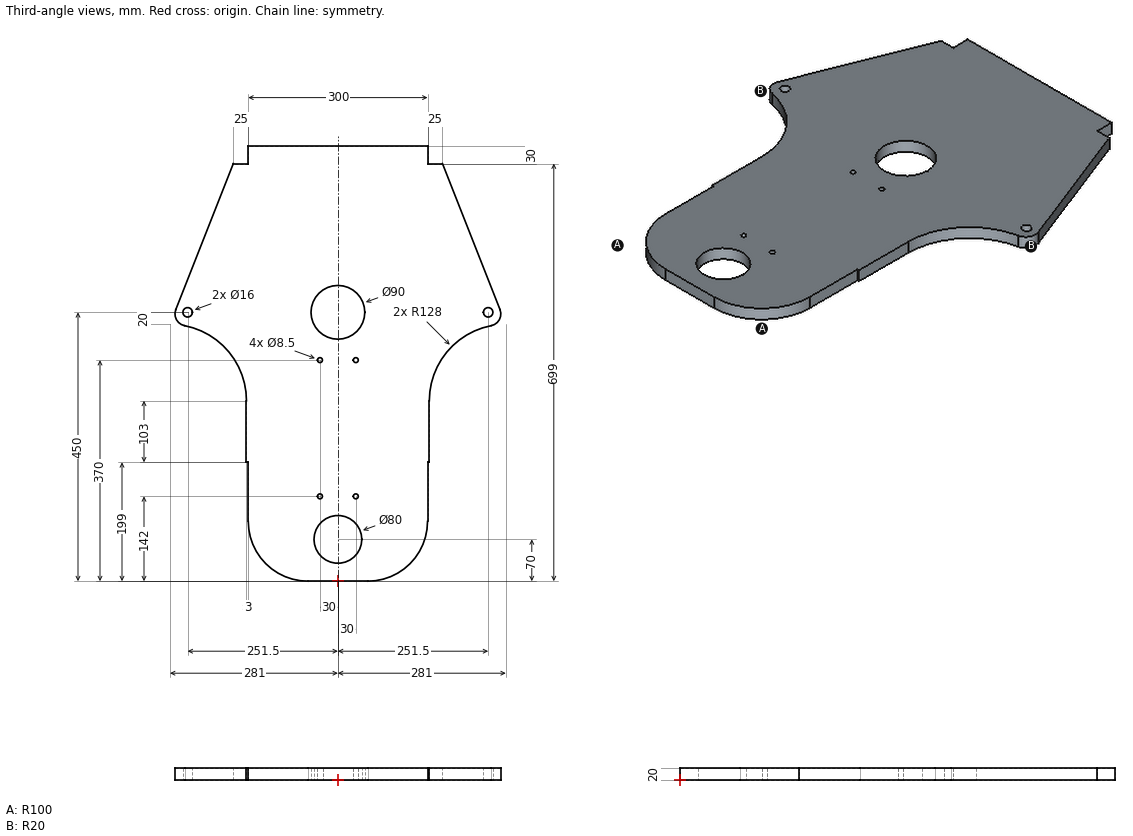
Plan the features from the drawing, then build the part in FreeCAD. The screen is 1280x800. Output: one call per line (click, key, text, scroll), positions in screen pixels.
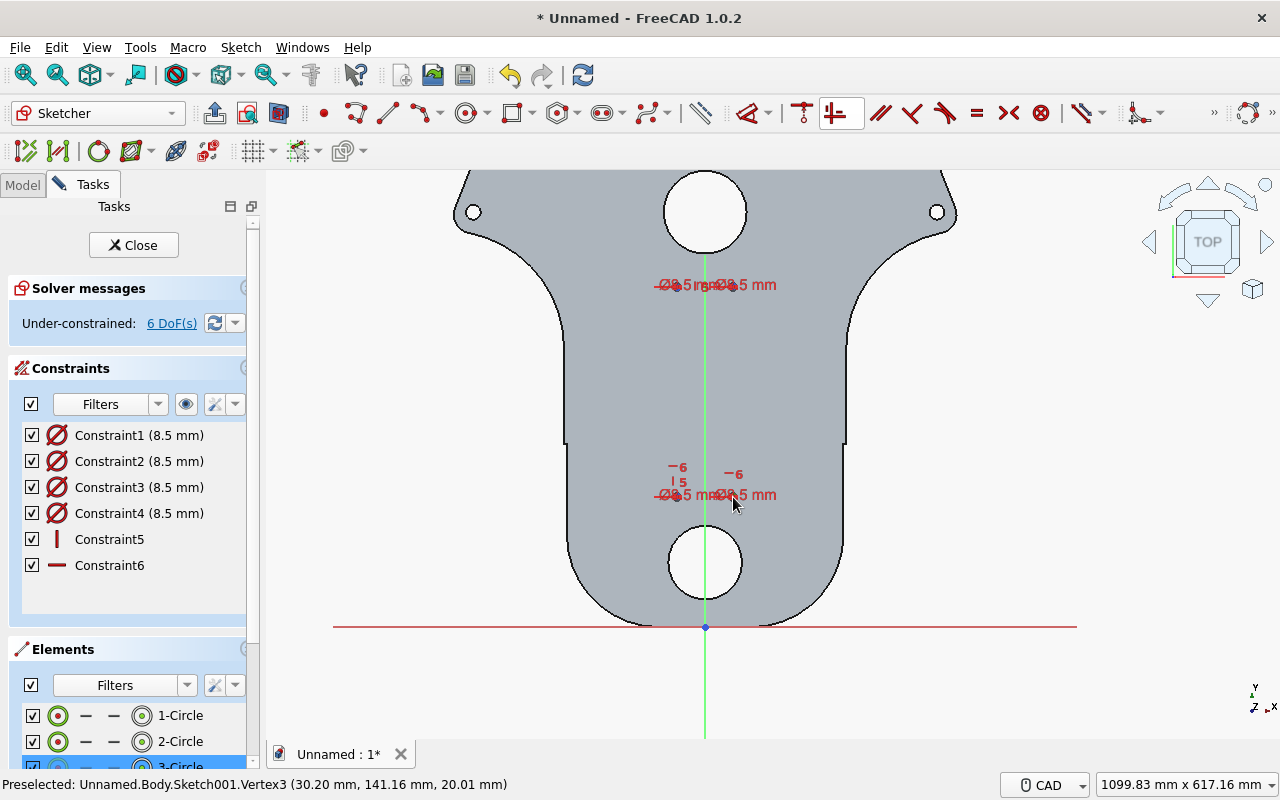
click(733, 287)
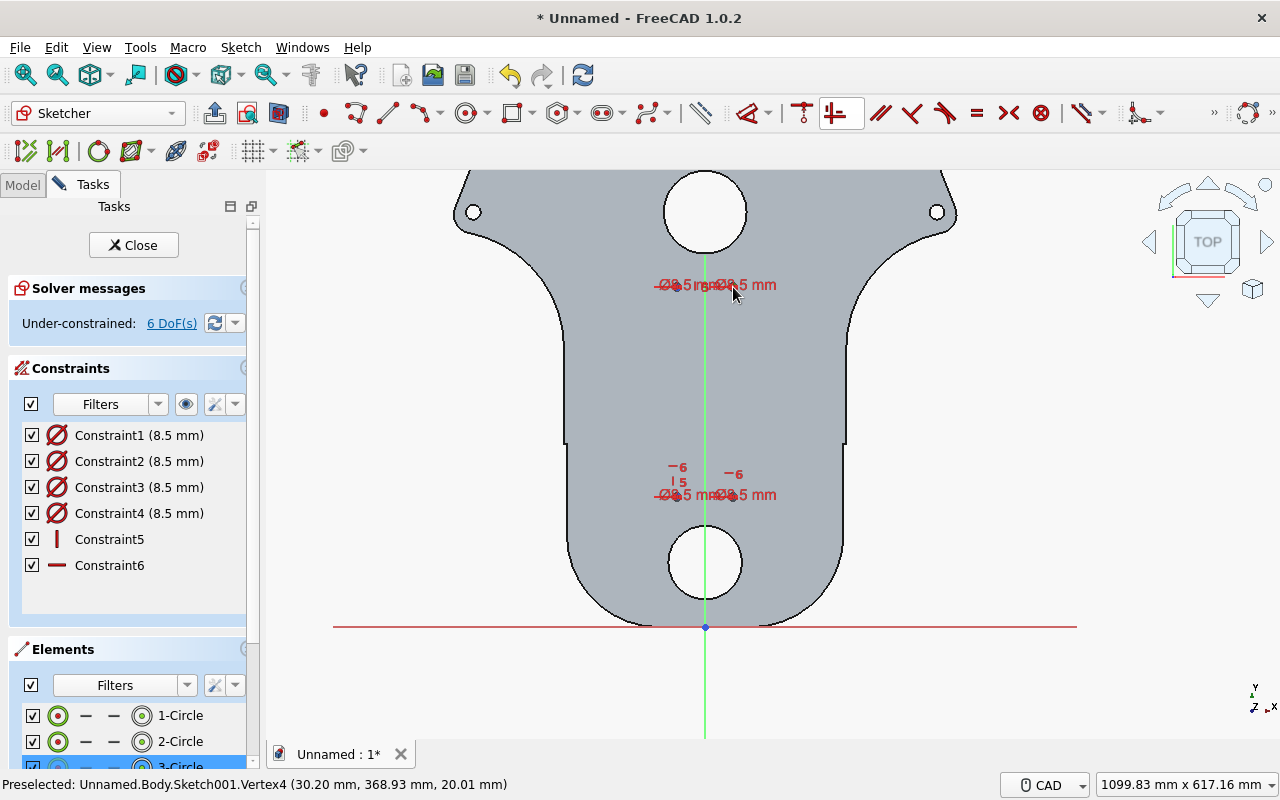
click(858, 114)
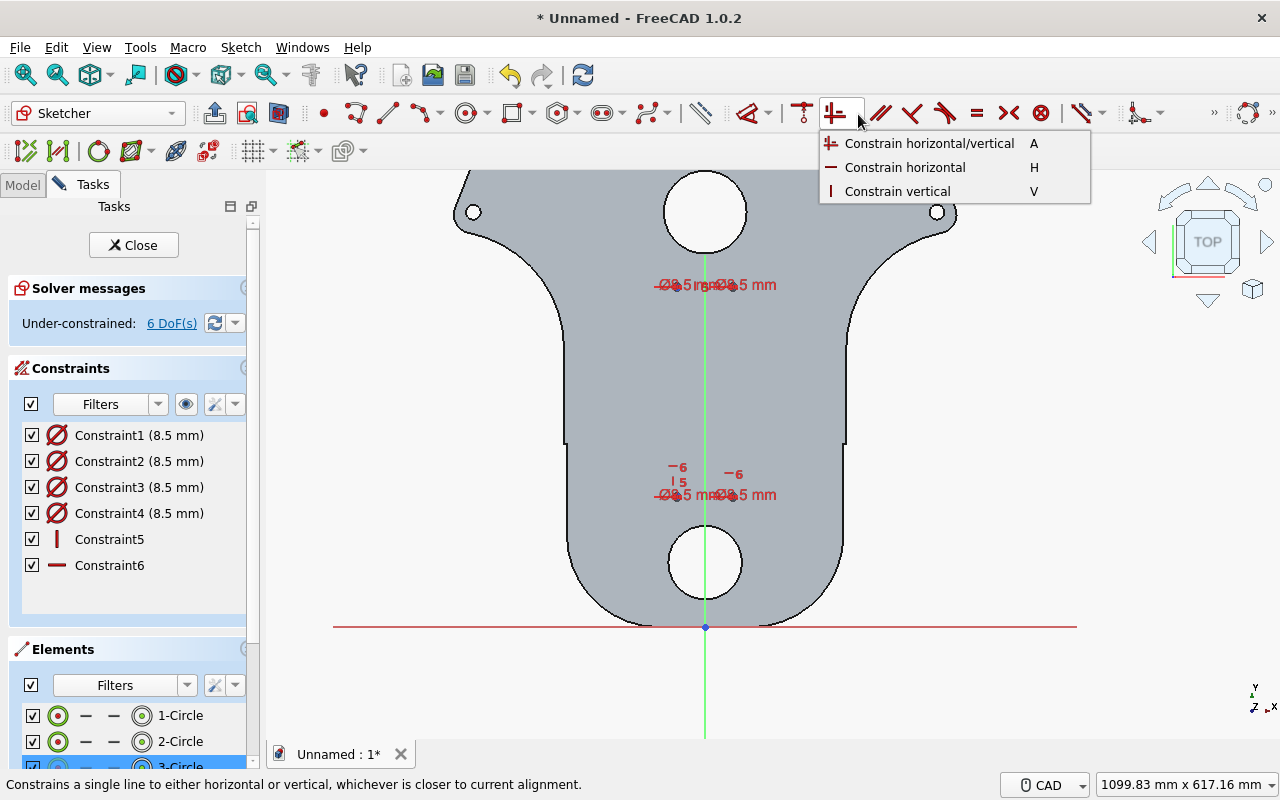
click(955, 191)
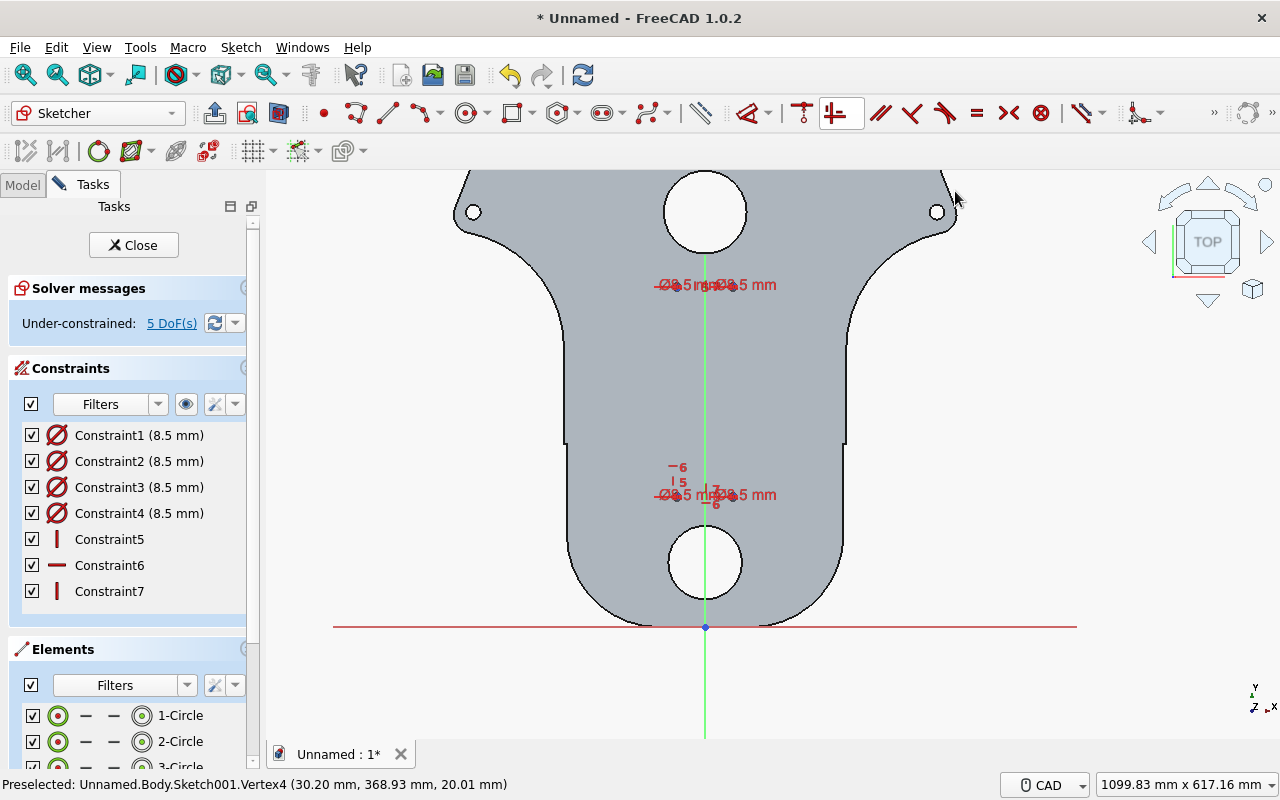
click(677, 287)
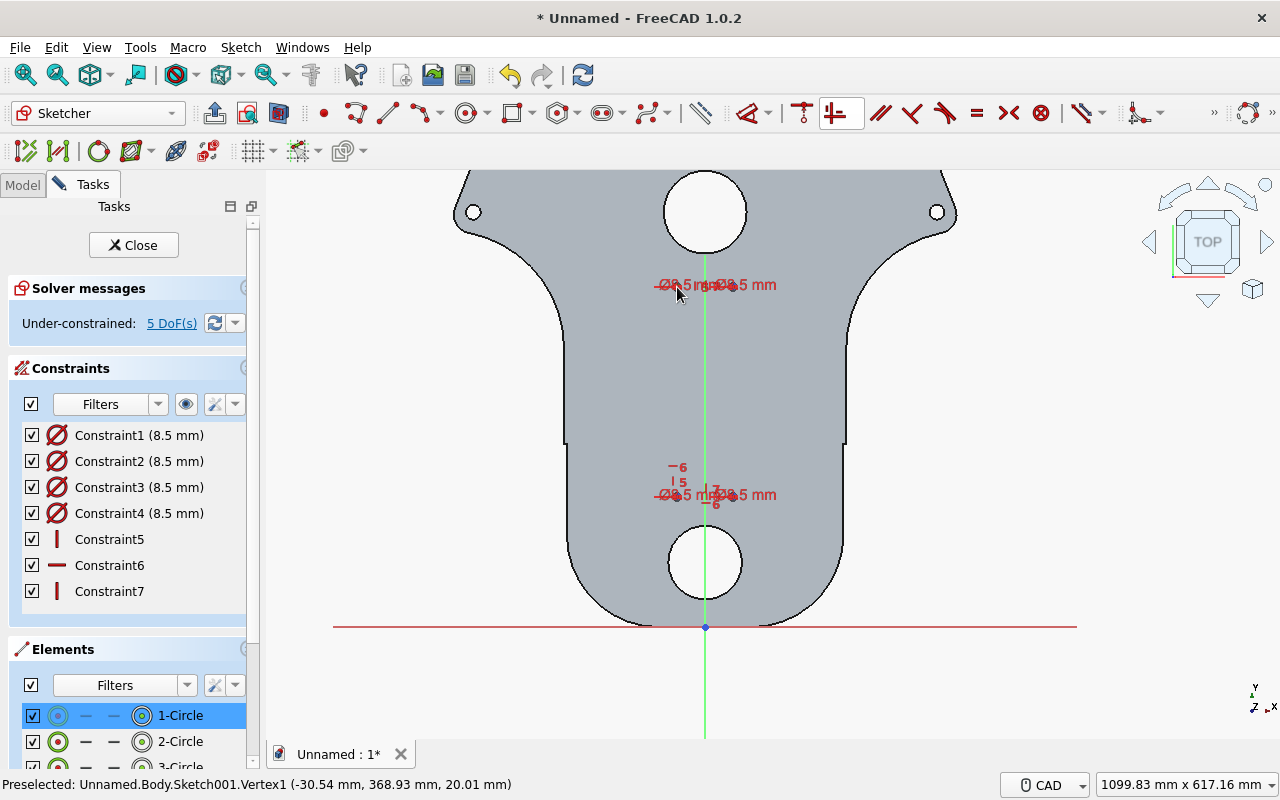
click(733, 287)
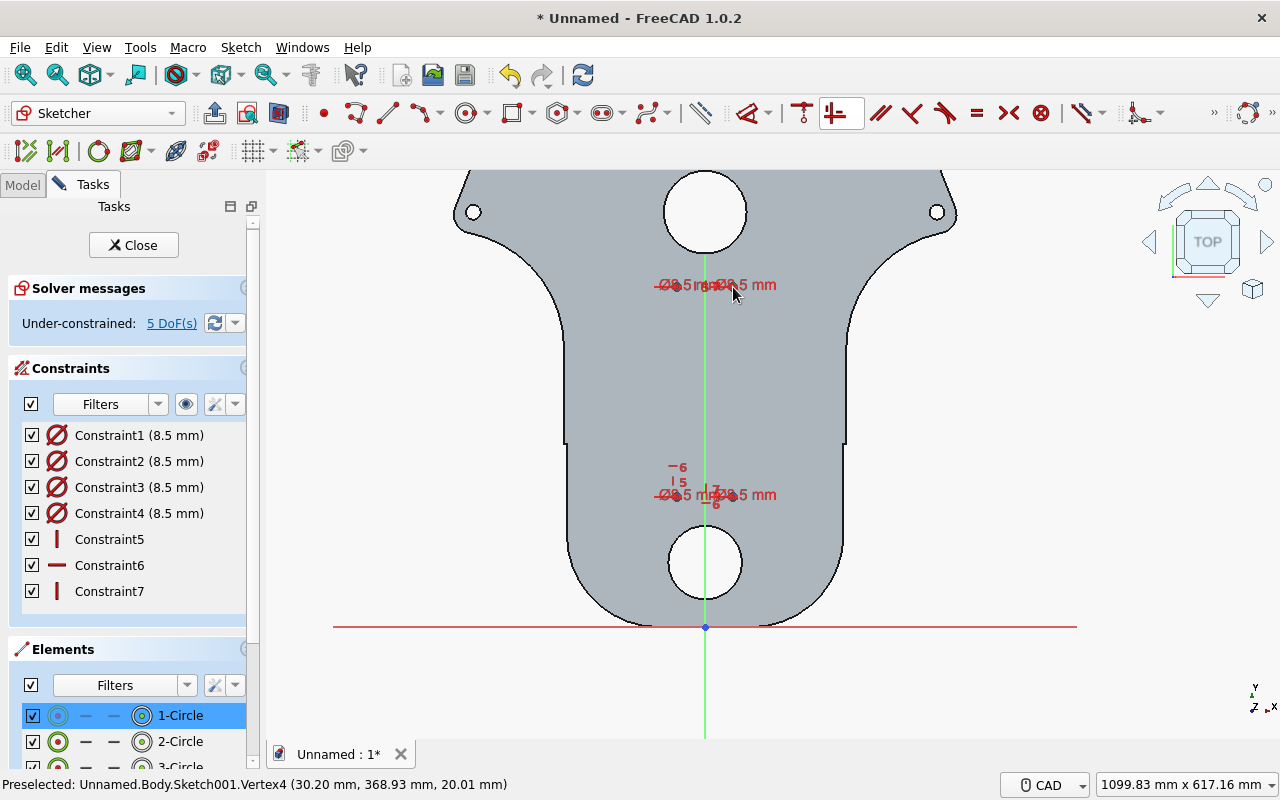
key(h)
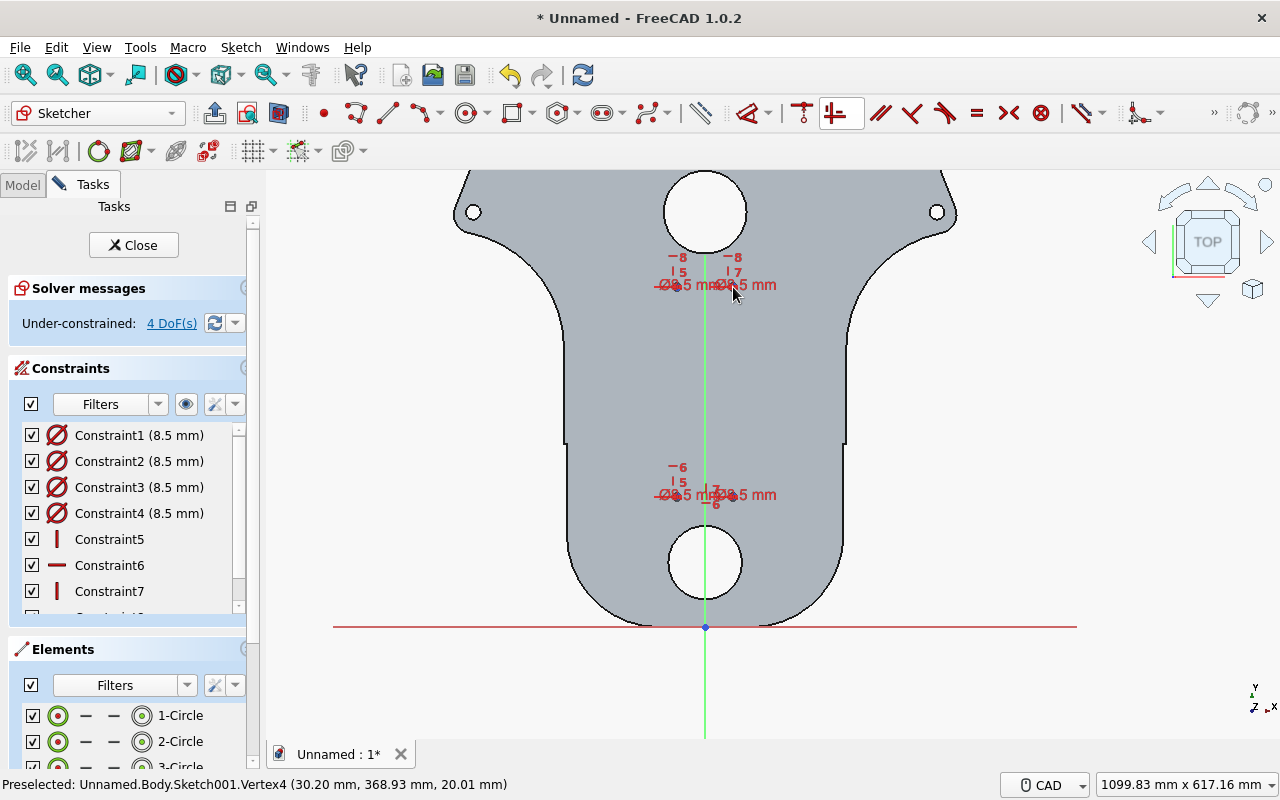
click(748, 114)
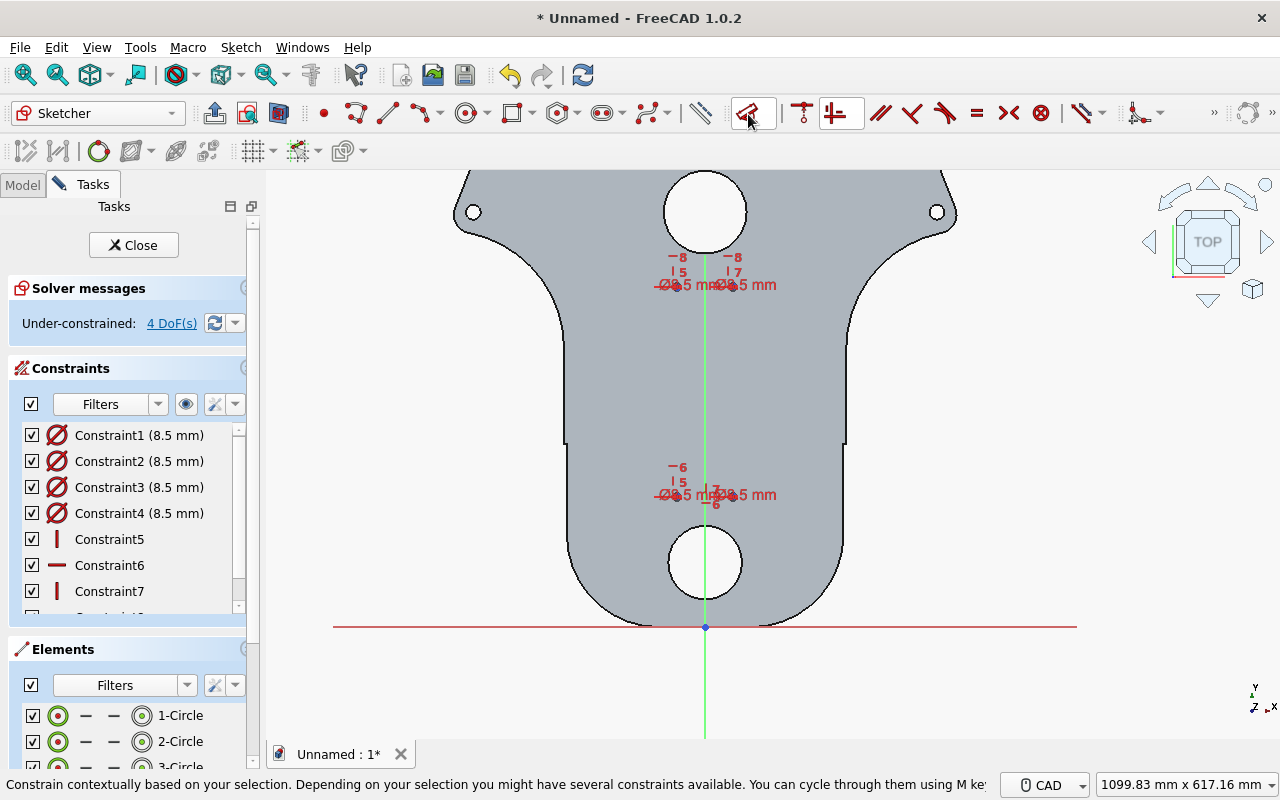
scroll(677, 287, up, 2)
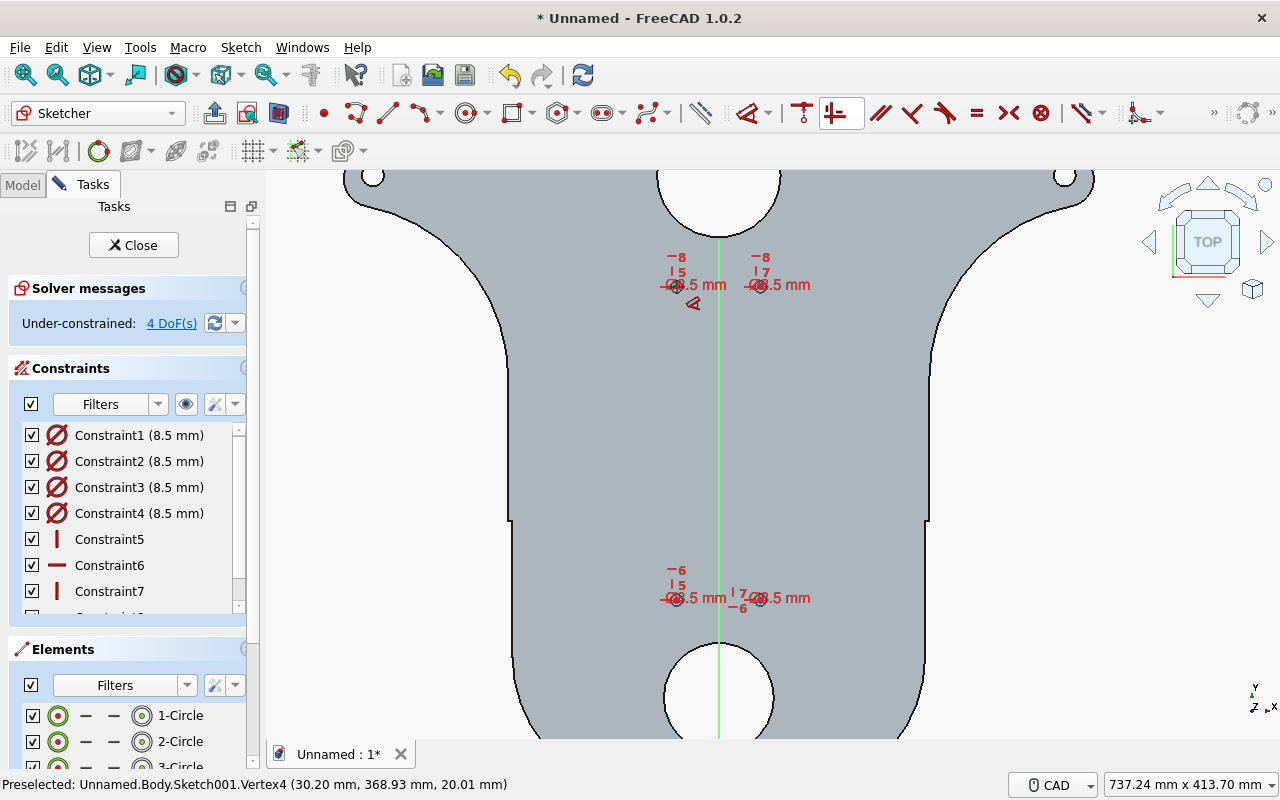
click(677, 287)
click(698, 253)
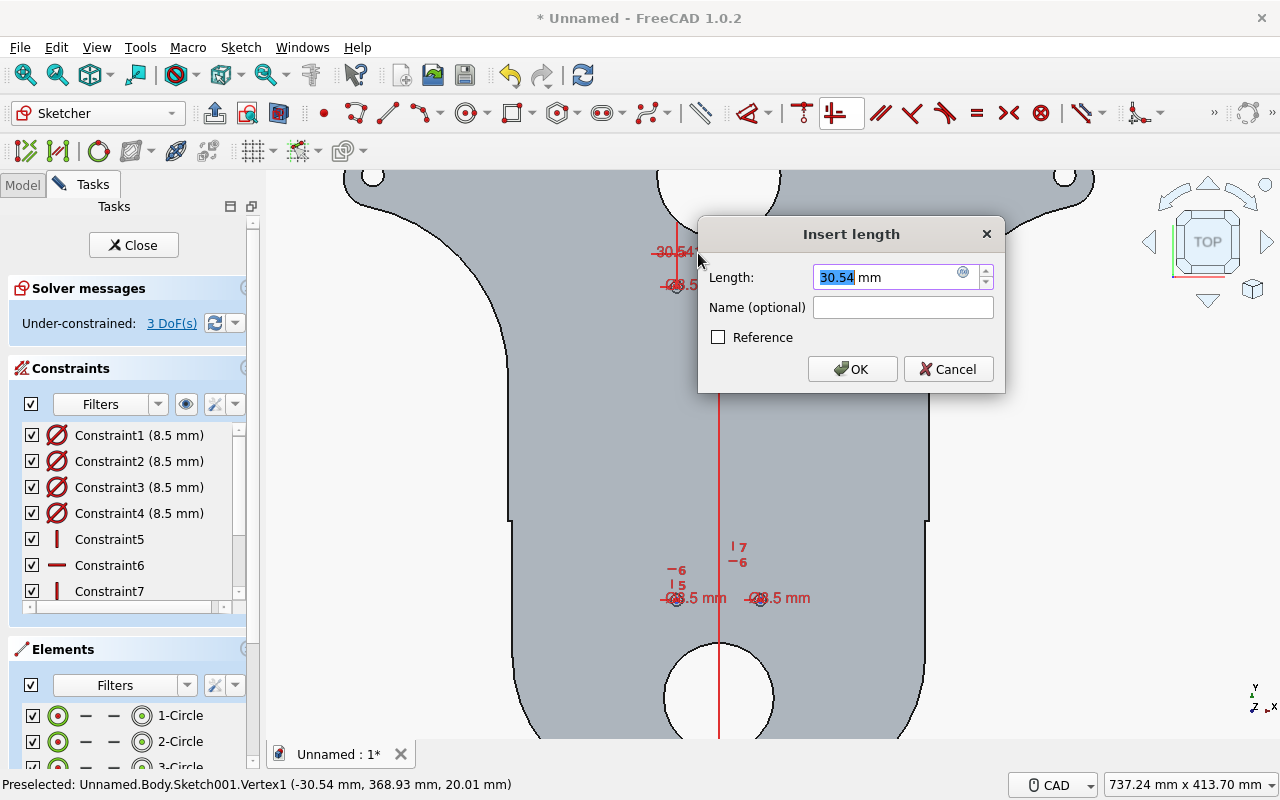
text(30)
key(Return)